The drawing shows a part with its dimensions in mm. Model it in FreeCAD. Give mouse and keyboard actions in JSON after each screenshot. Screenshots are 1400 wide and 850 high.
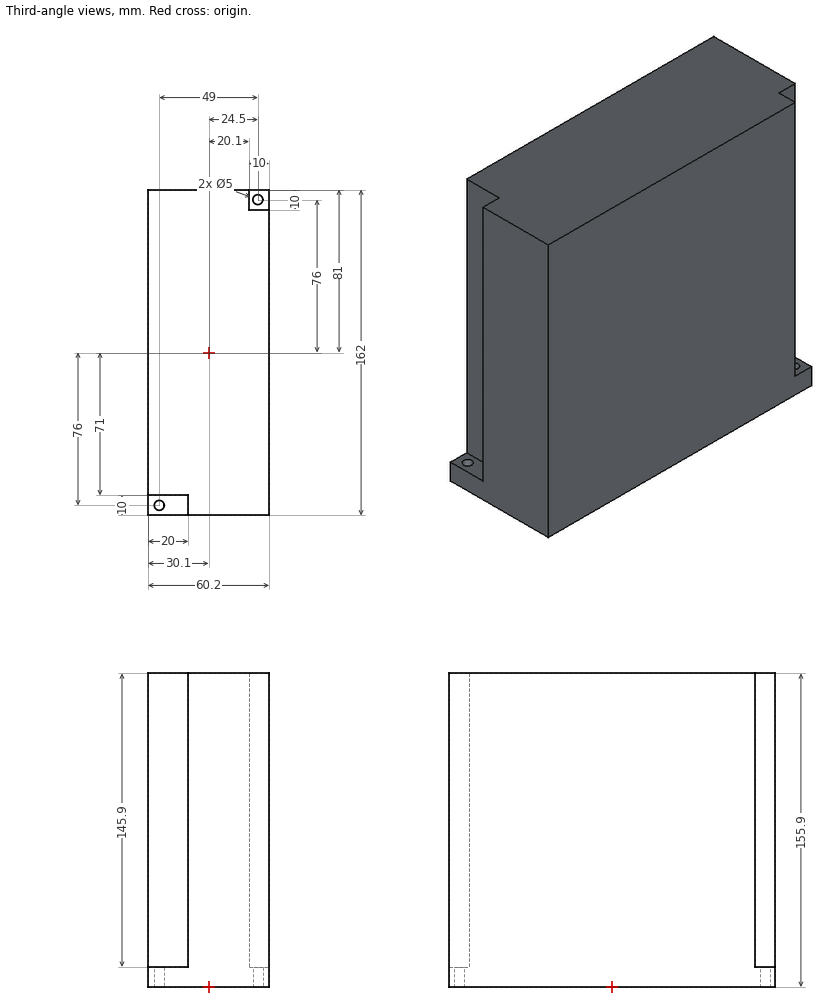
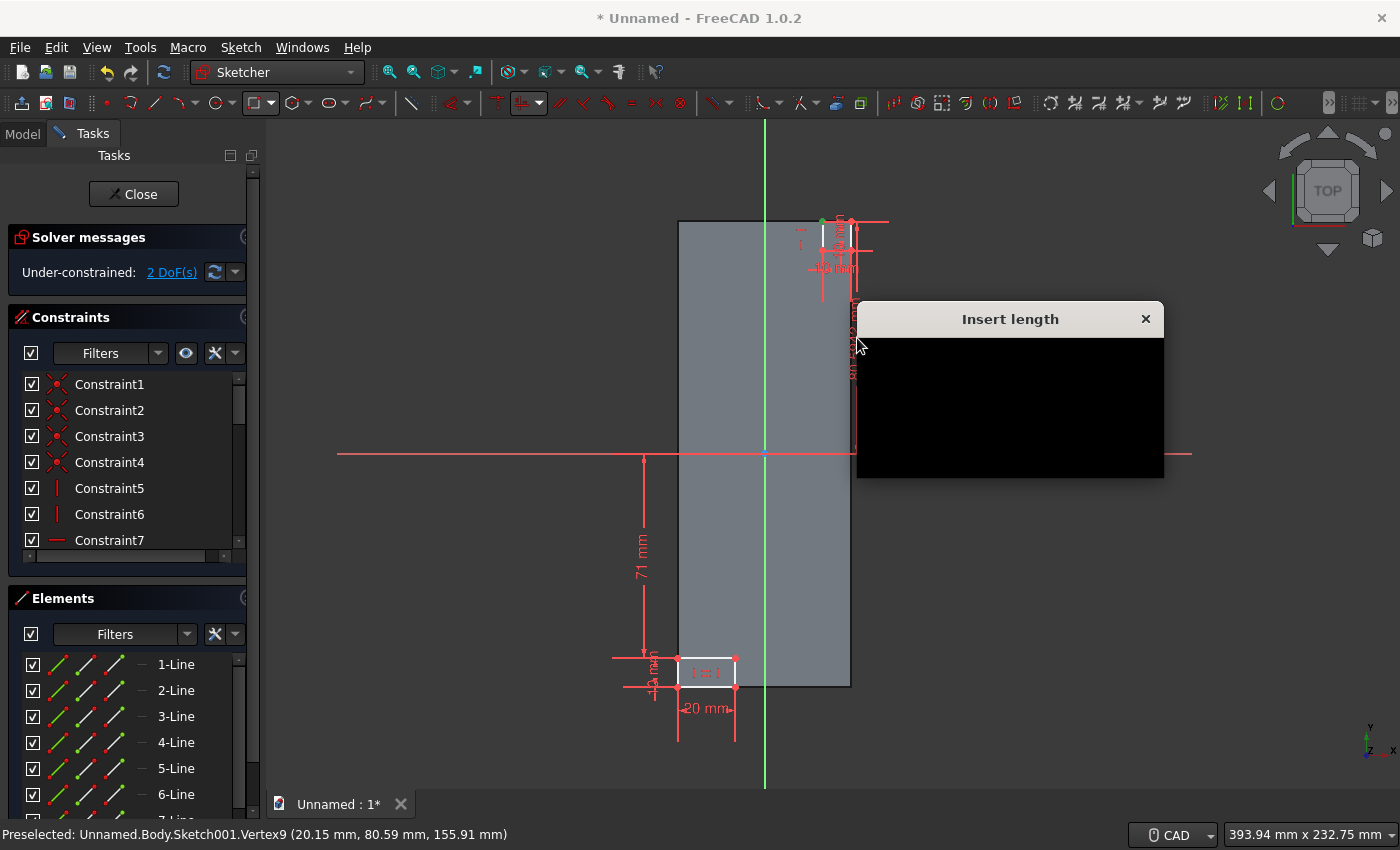
{"action": "type", "text": "81"}
{"action": "key", "text": "Return"}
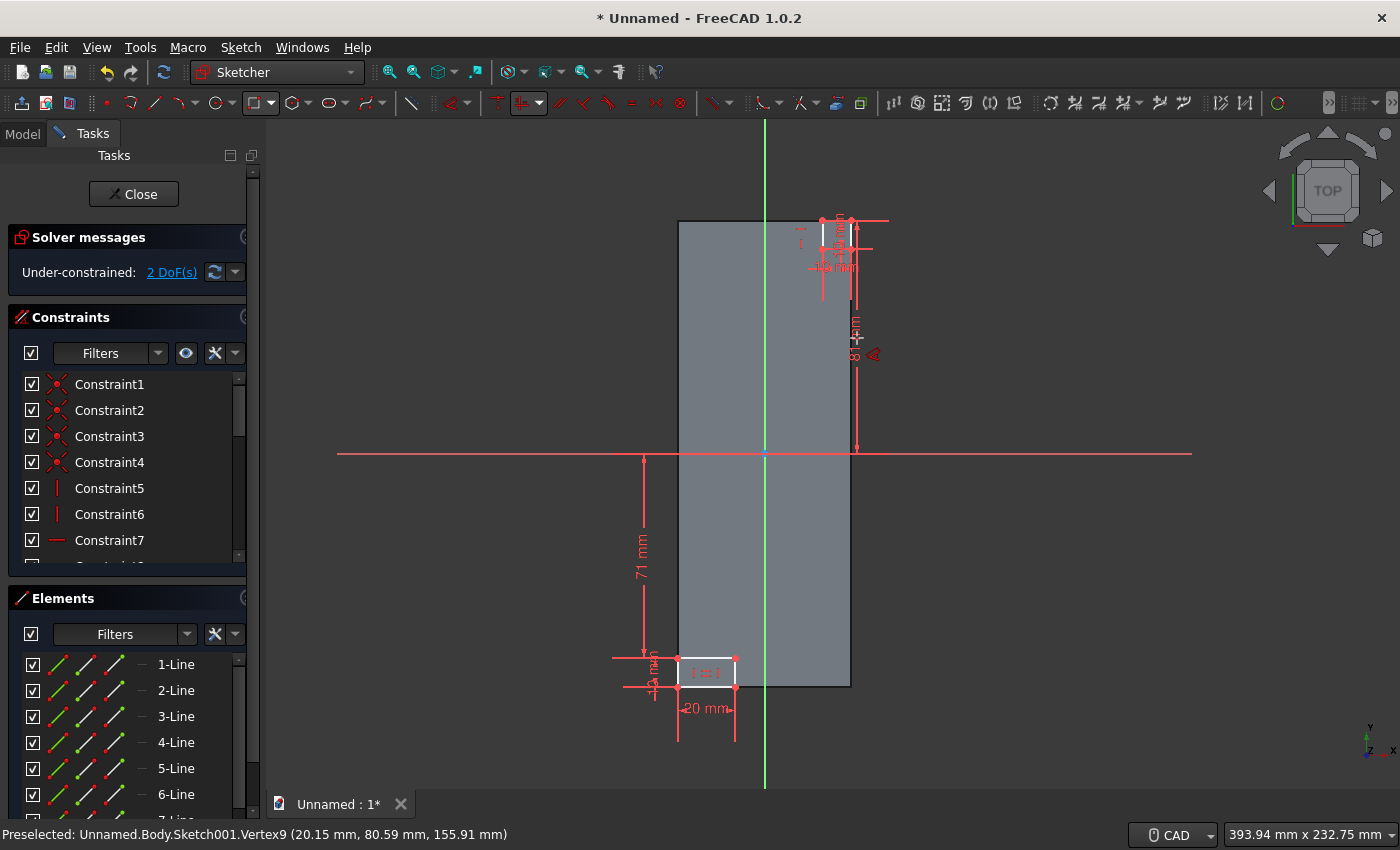
{"action": "left_click", "coordinate": [678, 658]}
{"action": "left_click", "coordinate": [721, 420]}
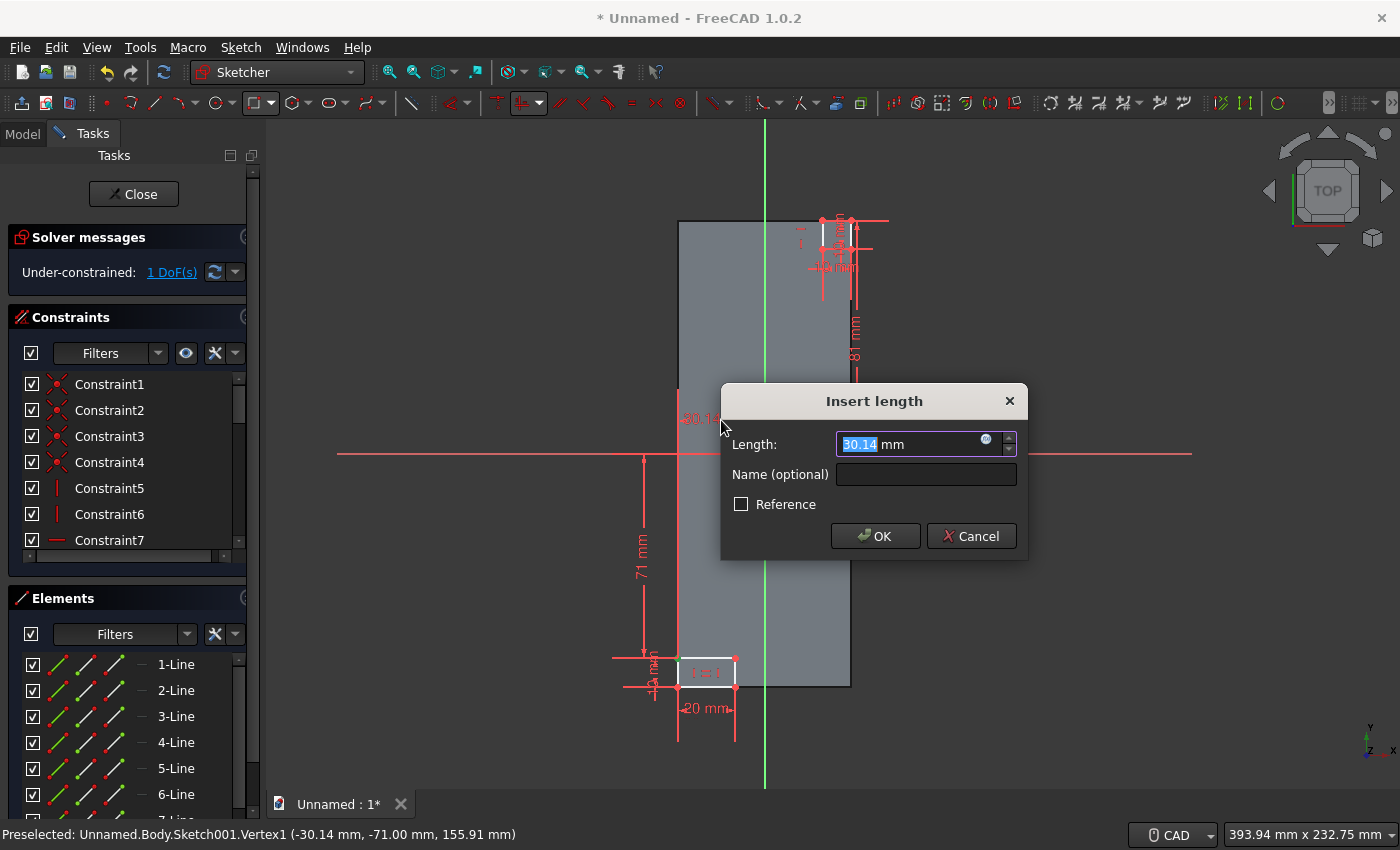
{"action": "type", "text": "30.1"}
{"action": "key", "text": "Return"}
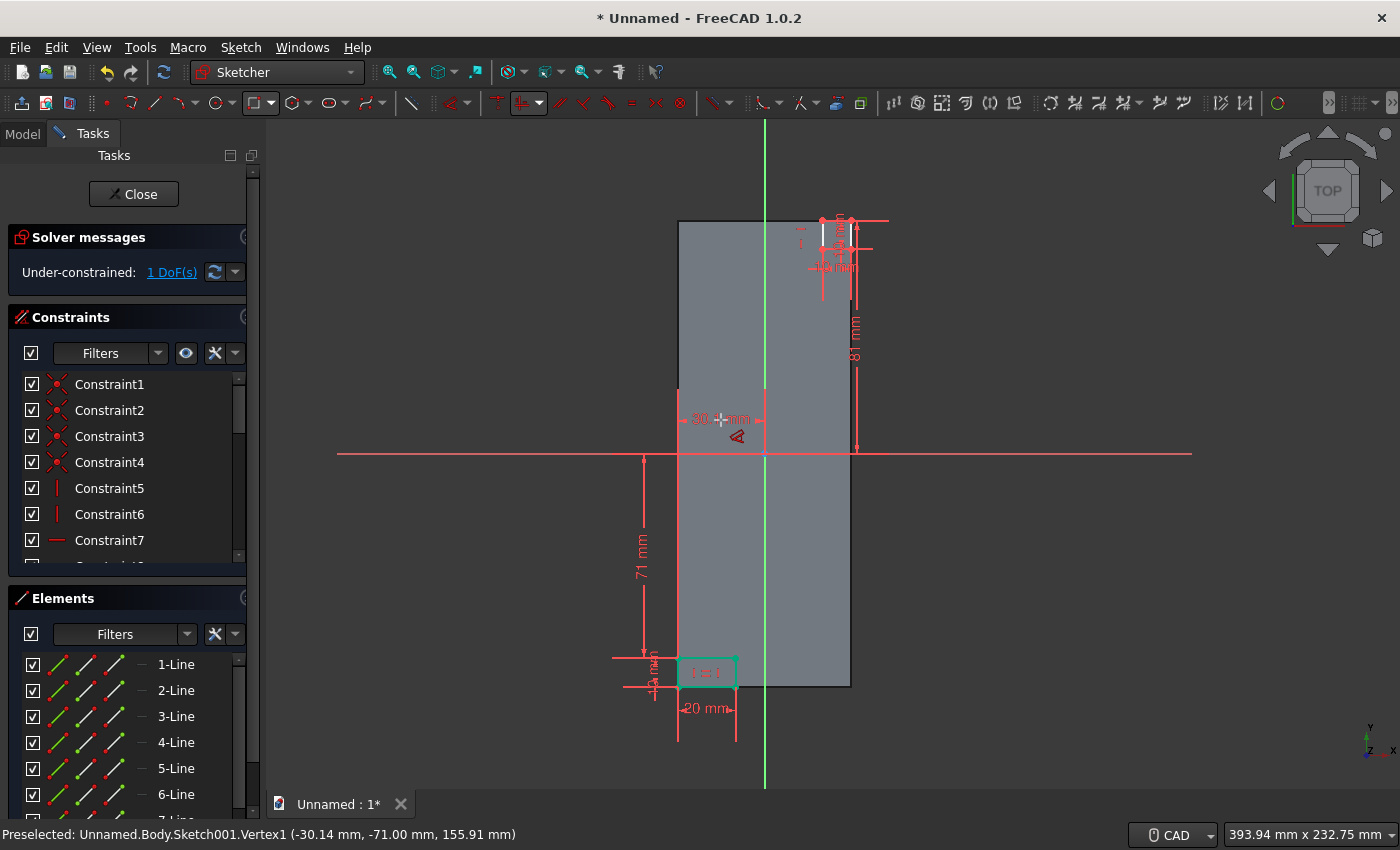
{"action": "left_click", "coordinate": [823, 221]}
{"action": "left_click", "coordinate": [794, 187]}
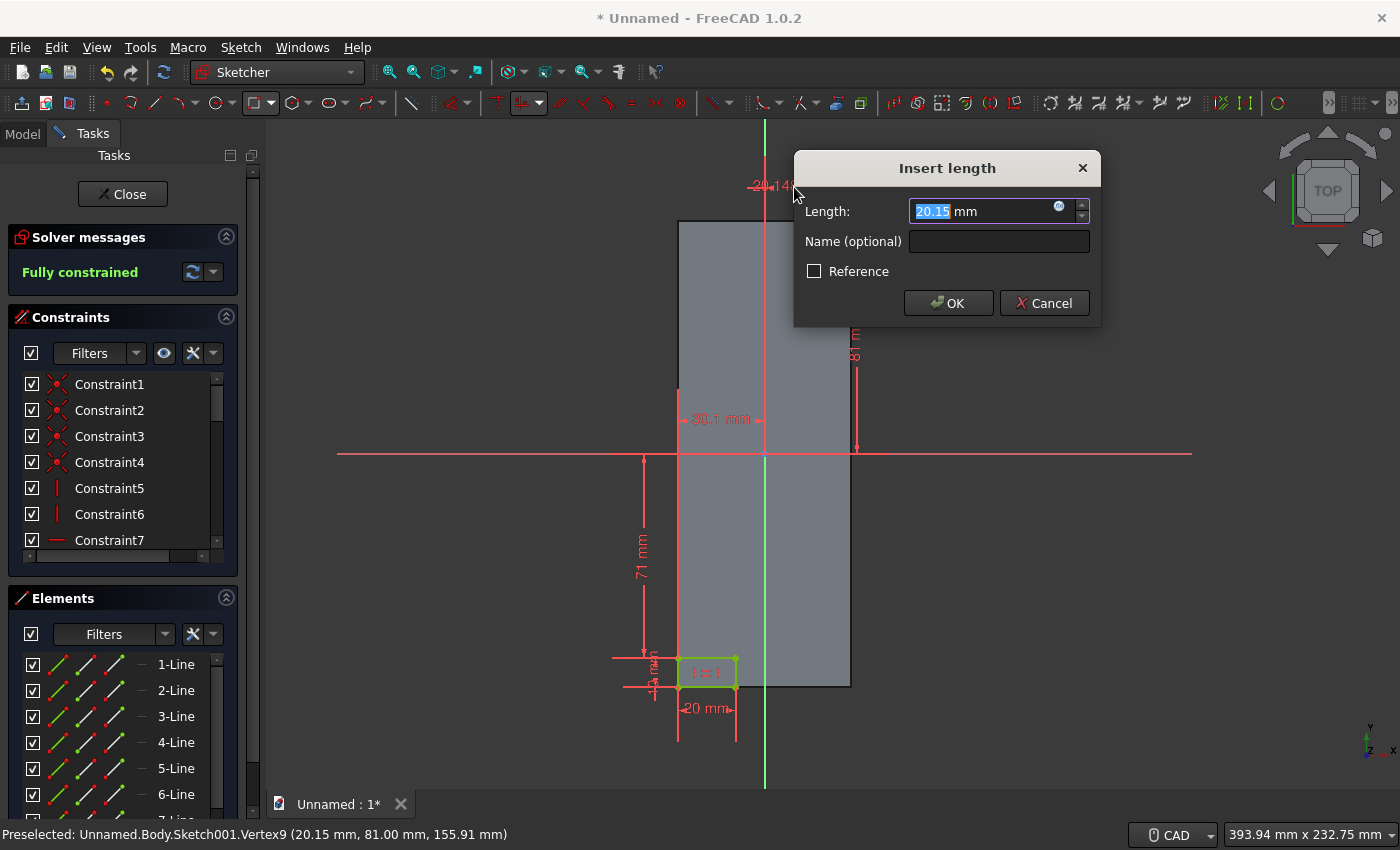
{"action": "type", "text": "20.1"}
{"action": "key", "text": "Return"}
{"action": "key", "text": "Escape"}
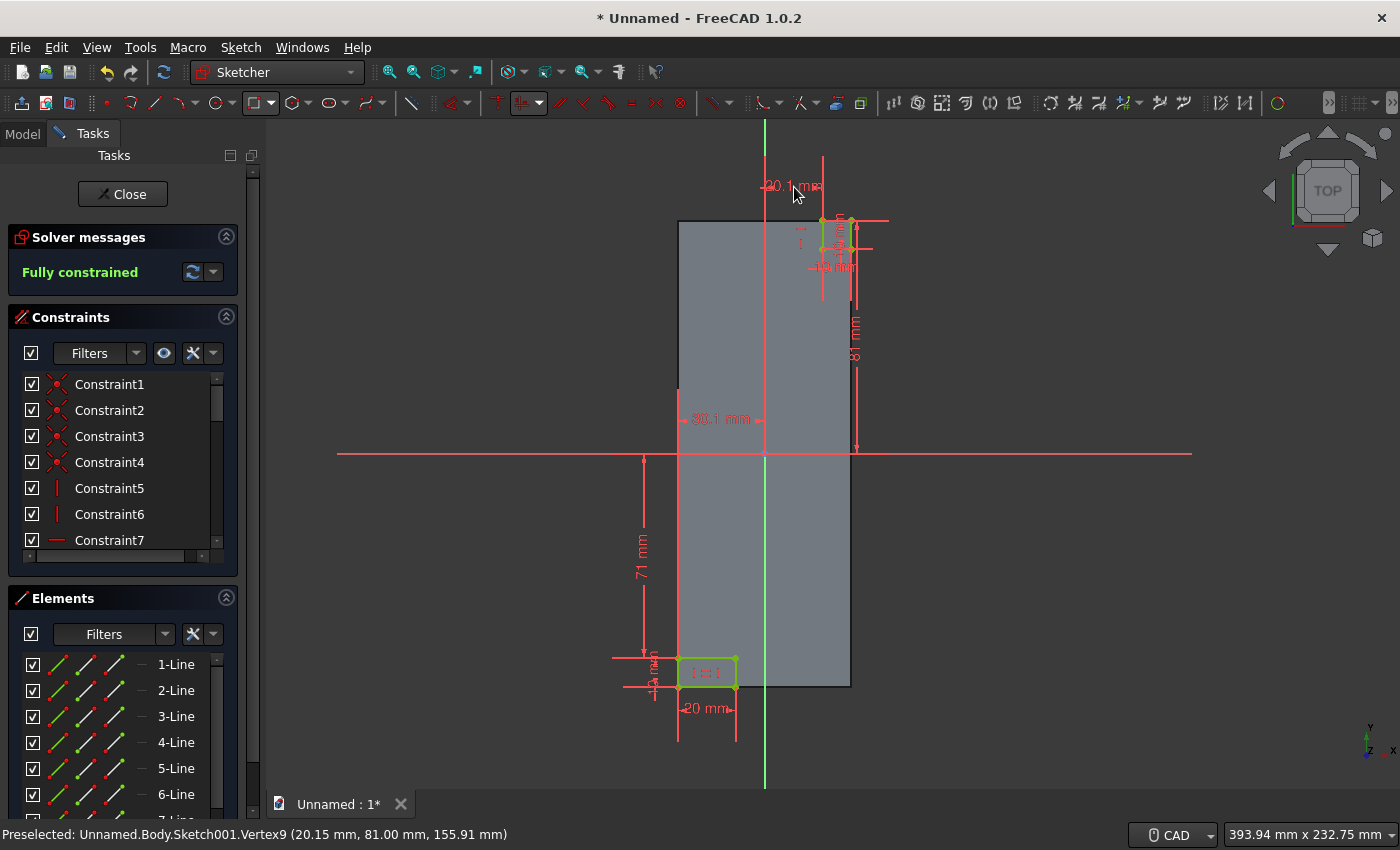
{"action": "left_click", "coordinate": [123, 194]}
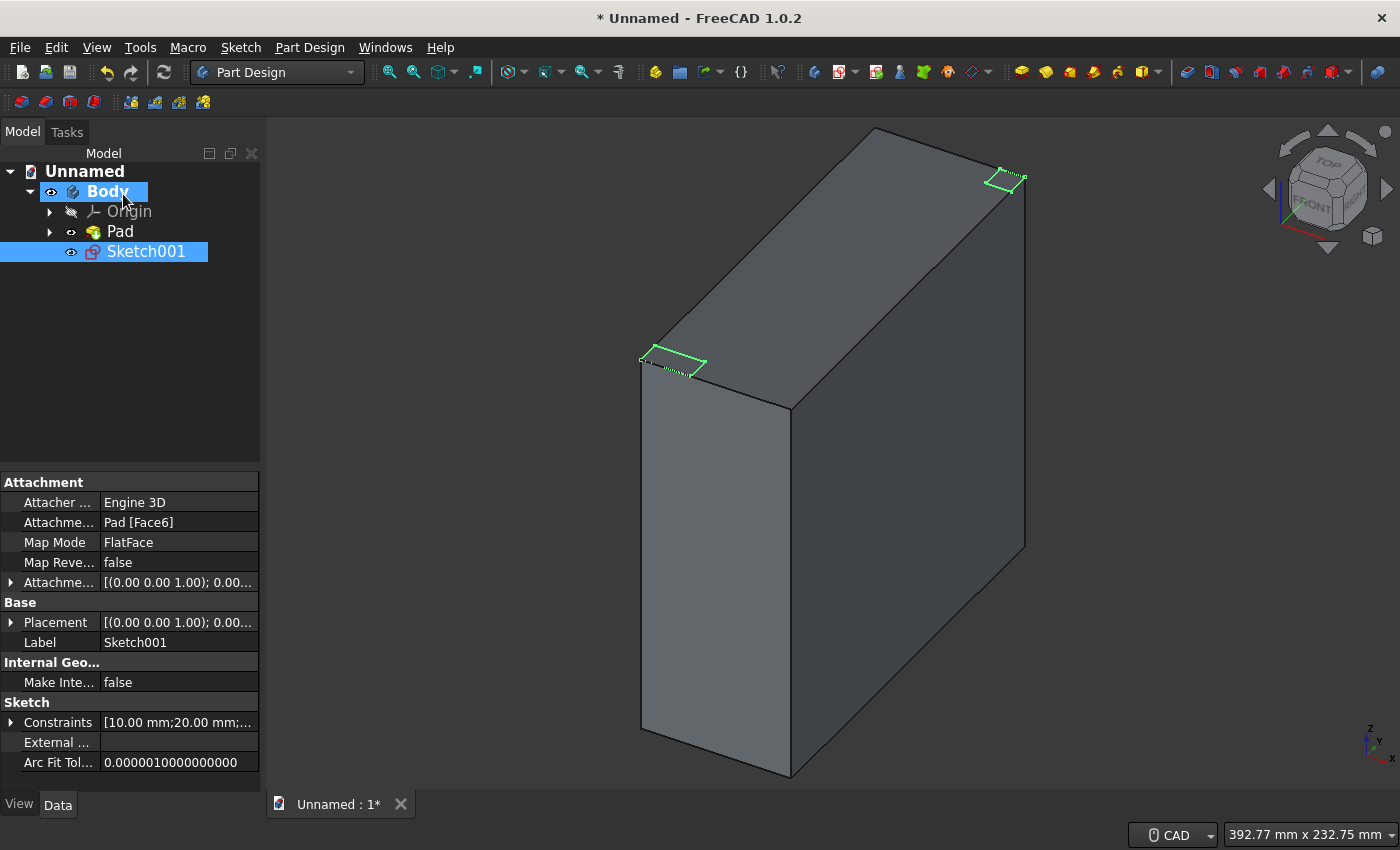
{"action": "left_click", "coordinate": [1188, 72]}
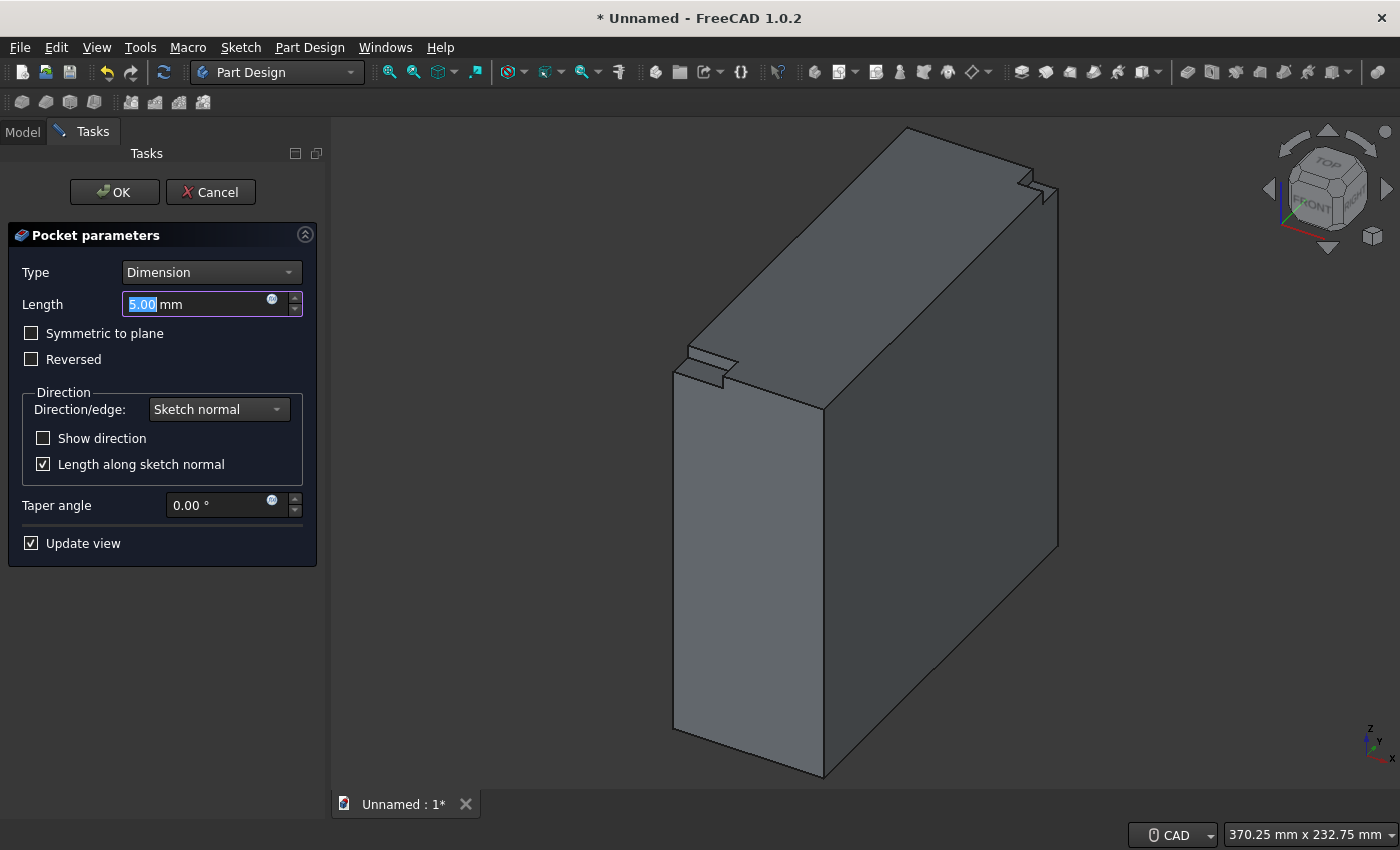
{"action": "type", "text": "145.9"}
{"action": "key", "text": "Tab"}